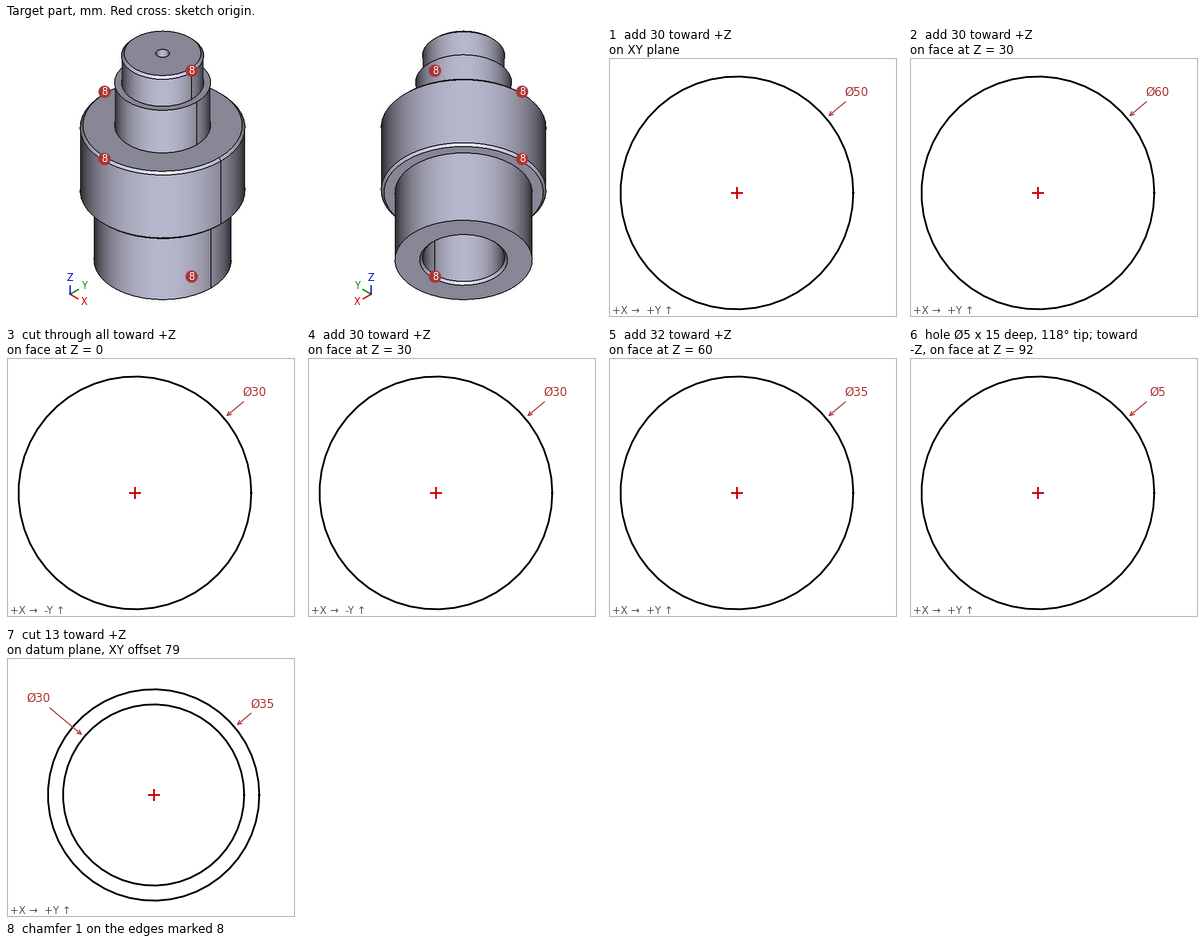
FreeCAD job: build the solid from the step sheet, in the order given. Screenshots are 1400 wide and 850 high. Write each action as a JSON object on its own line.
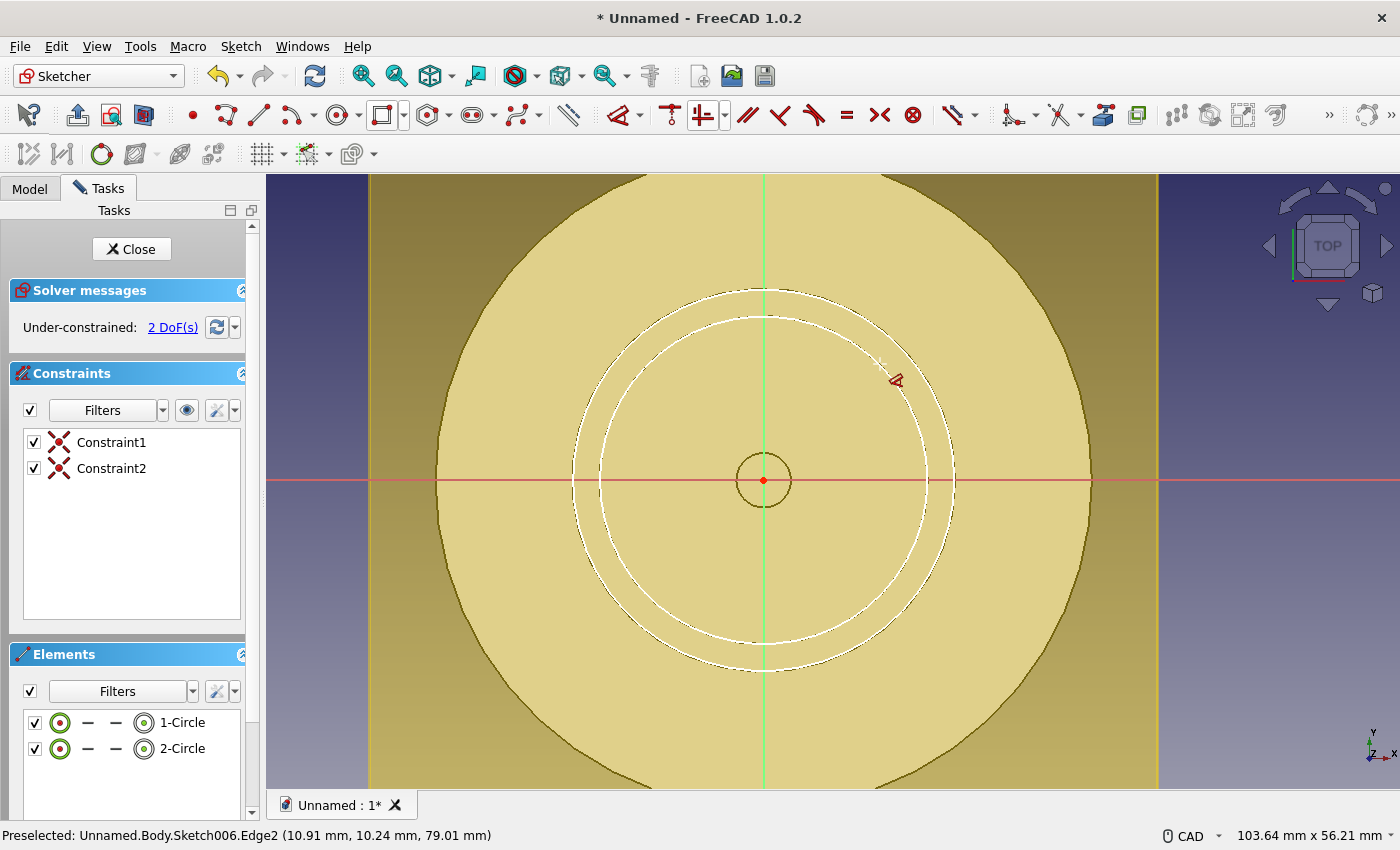
{"action": "left_click", "coordinate": [898, 345]}
{"action": "left_click", "coordinate": [921, 322]}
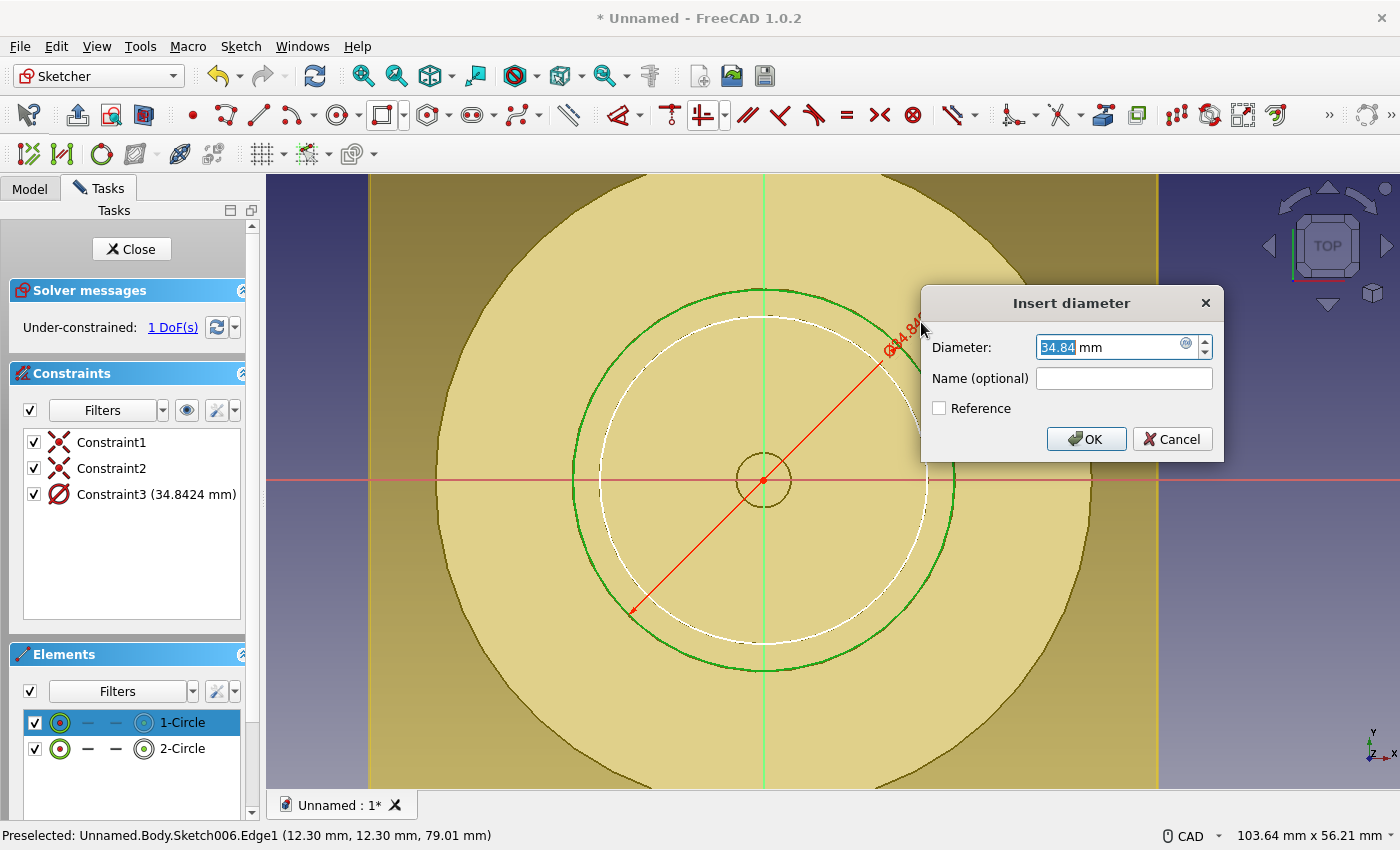
{"action": "type", "text": "35"}
{"action": "key", "text": "Return"}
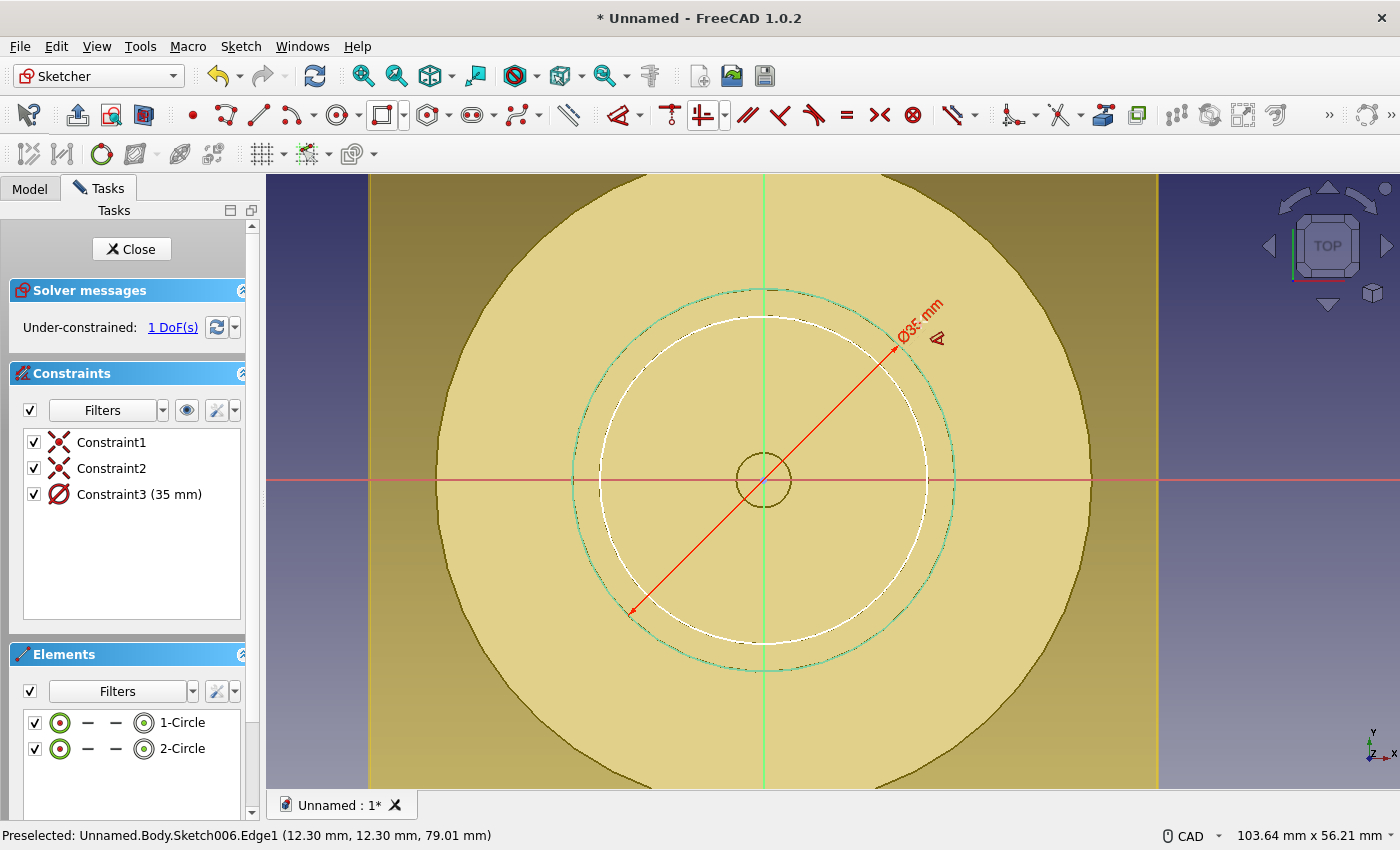
{"action": "left_click", "coordinate": [879, 364]}
{"action": "left_click", "coordinate": [973, 418]}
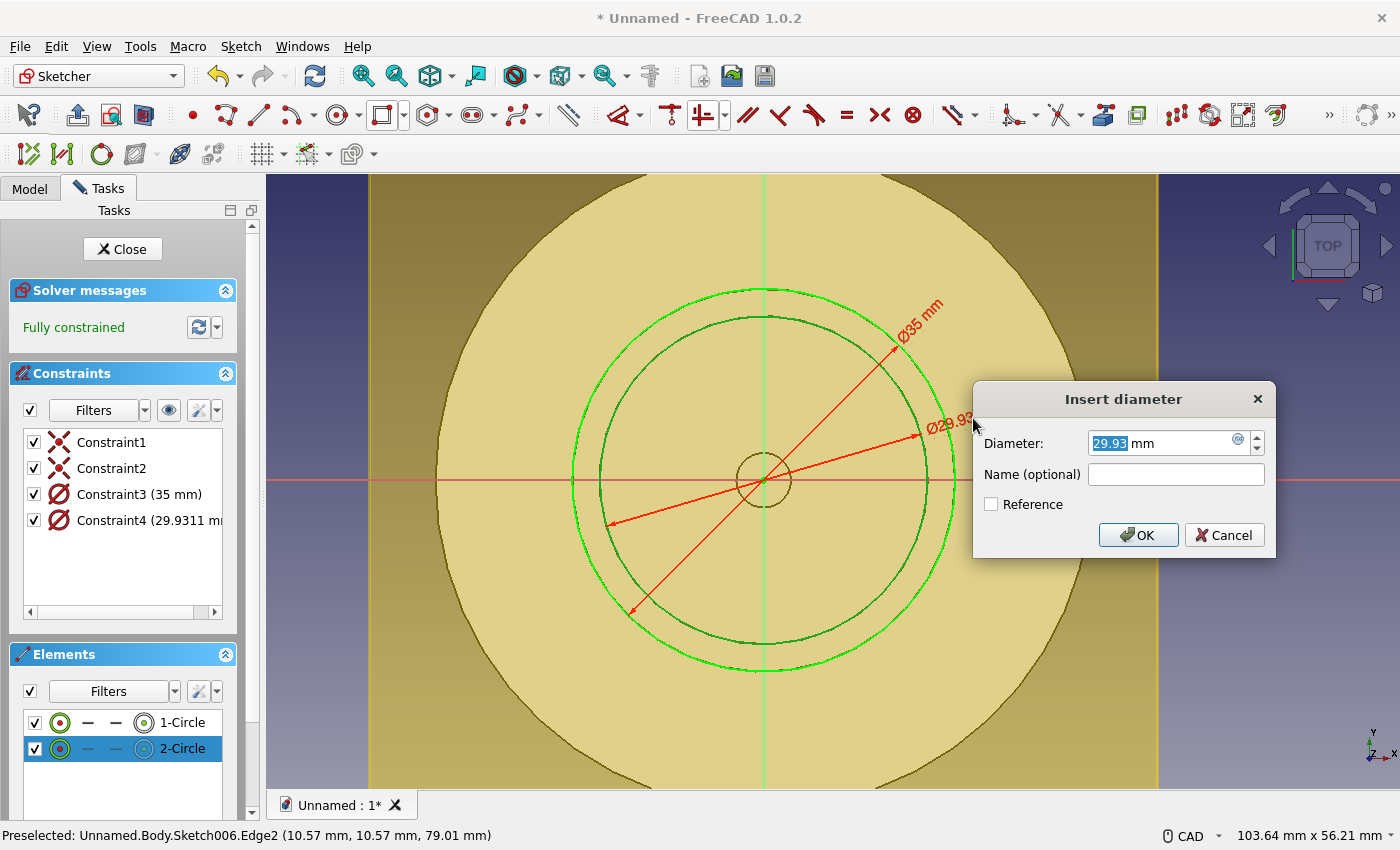
{"action": "type", "text": "30"}
{"action": "key", "text": "Return"}
{"action": "key", "text": "Escape"}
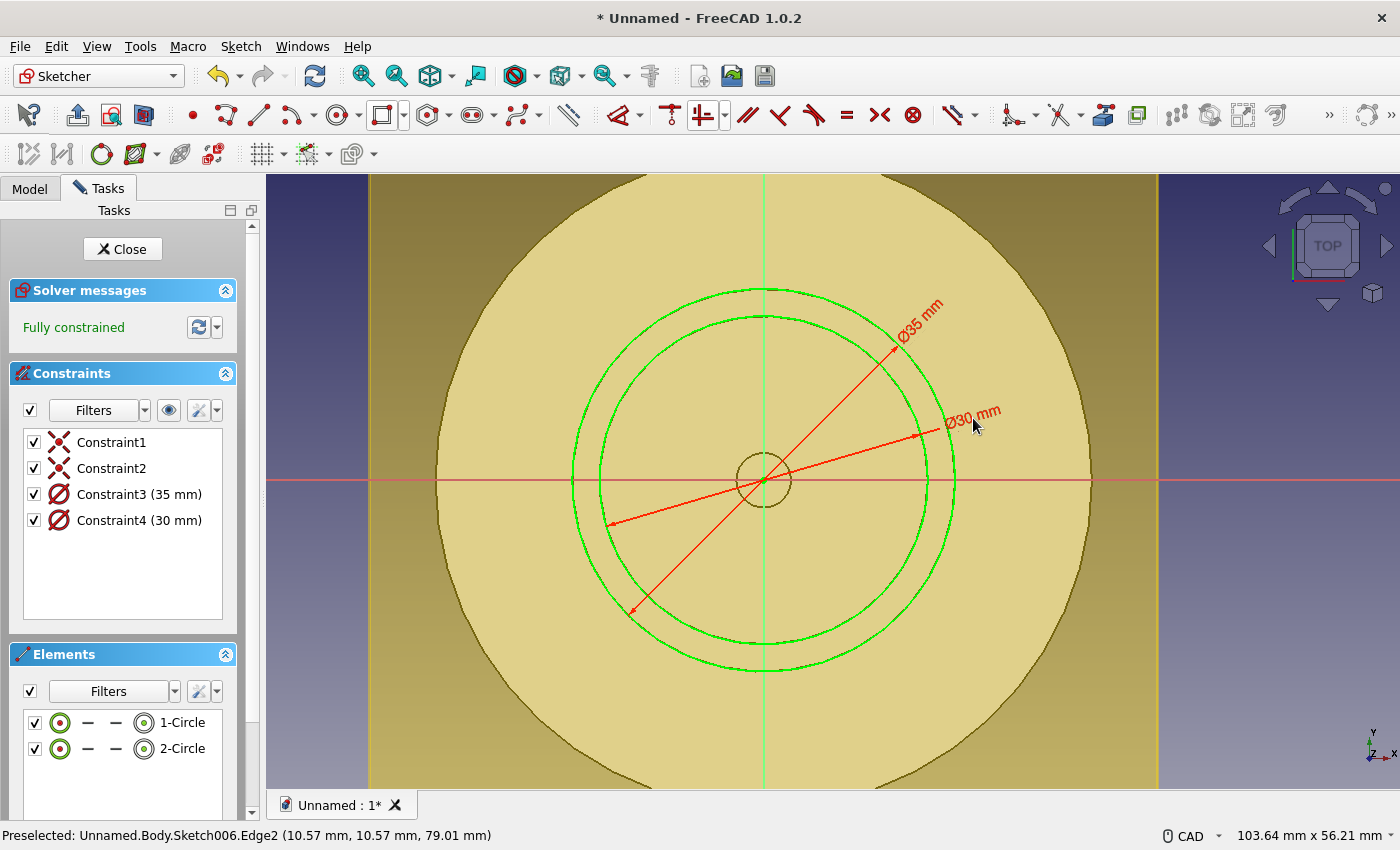
{"action": "left_click", "coordinate": [123, 249]}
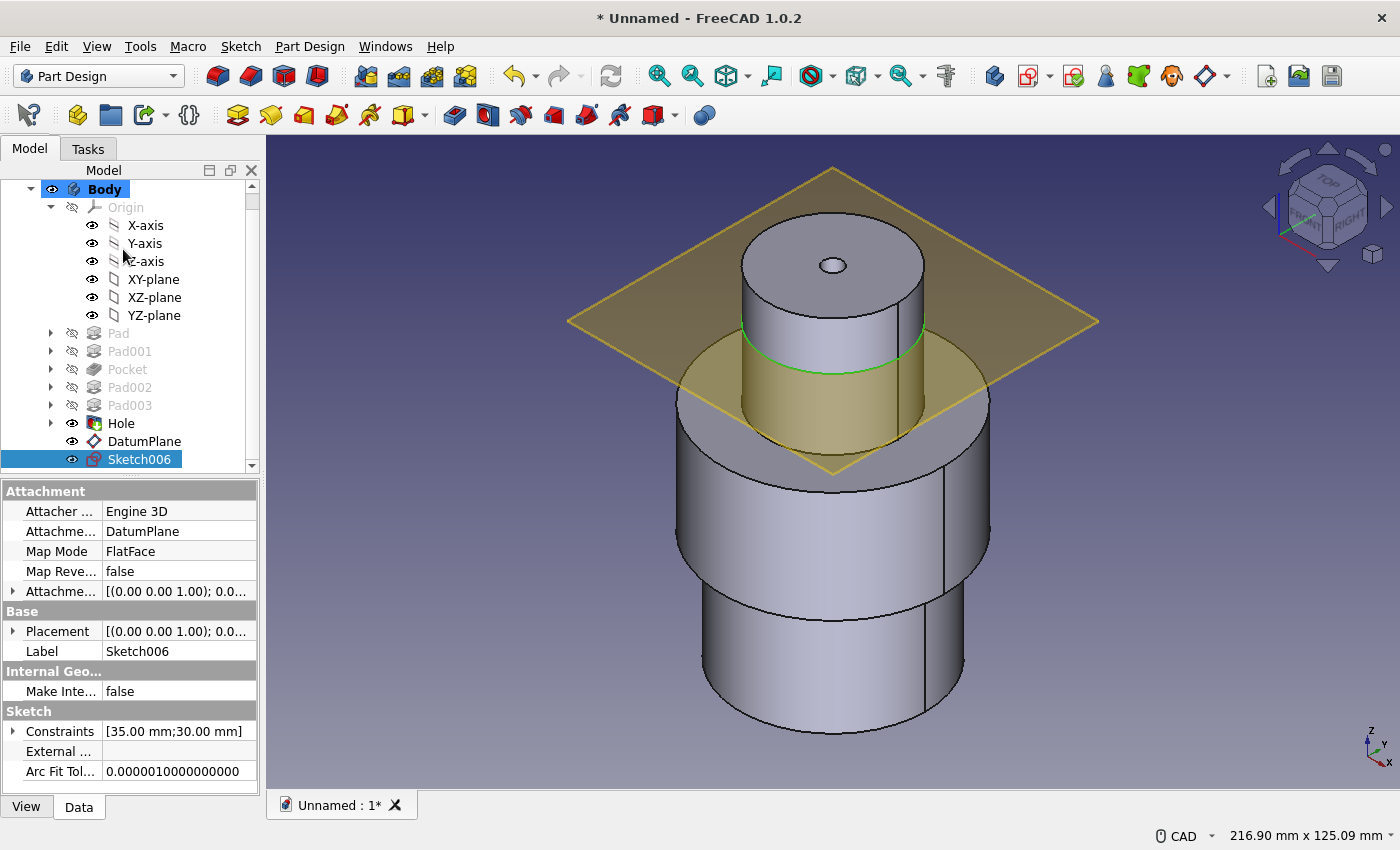
{"action": "left_click", "coordinate": [455, 116]}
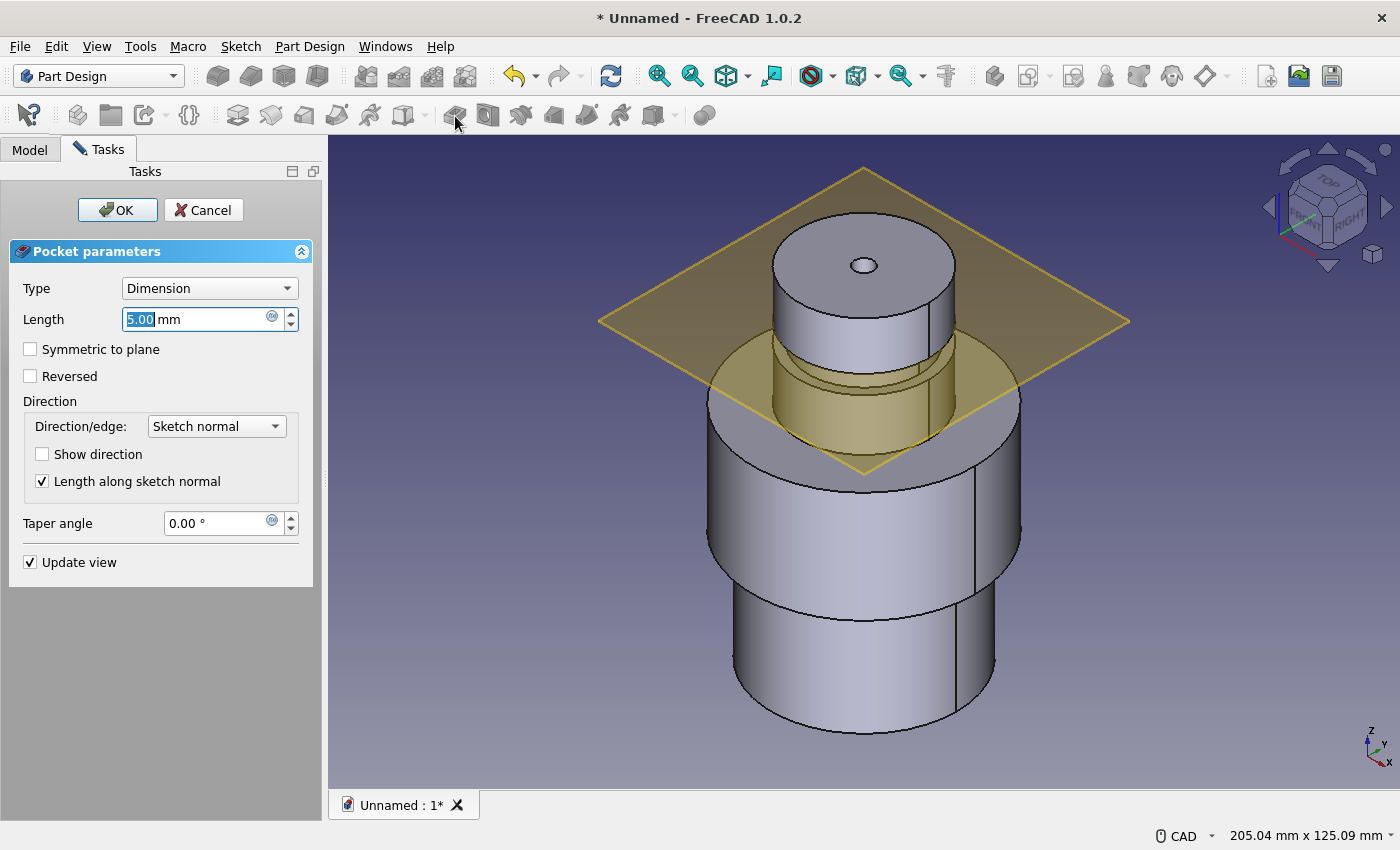
{"action": "type", "text": "13"}
{"action": "key", "text": "Tab"}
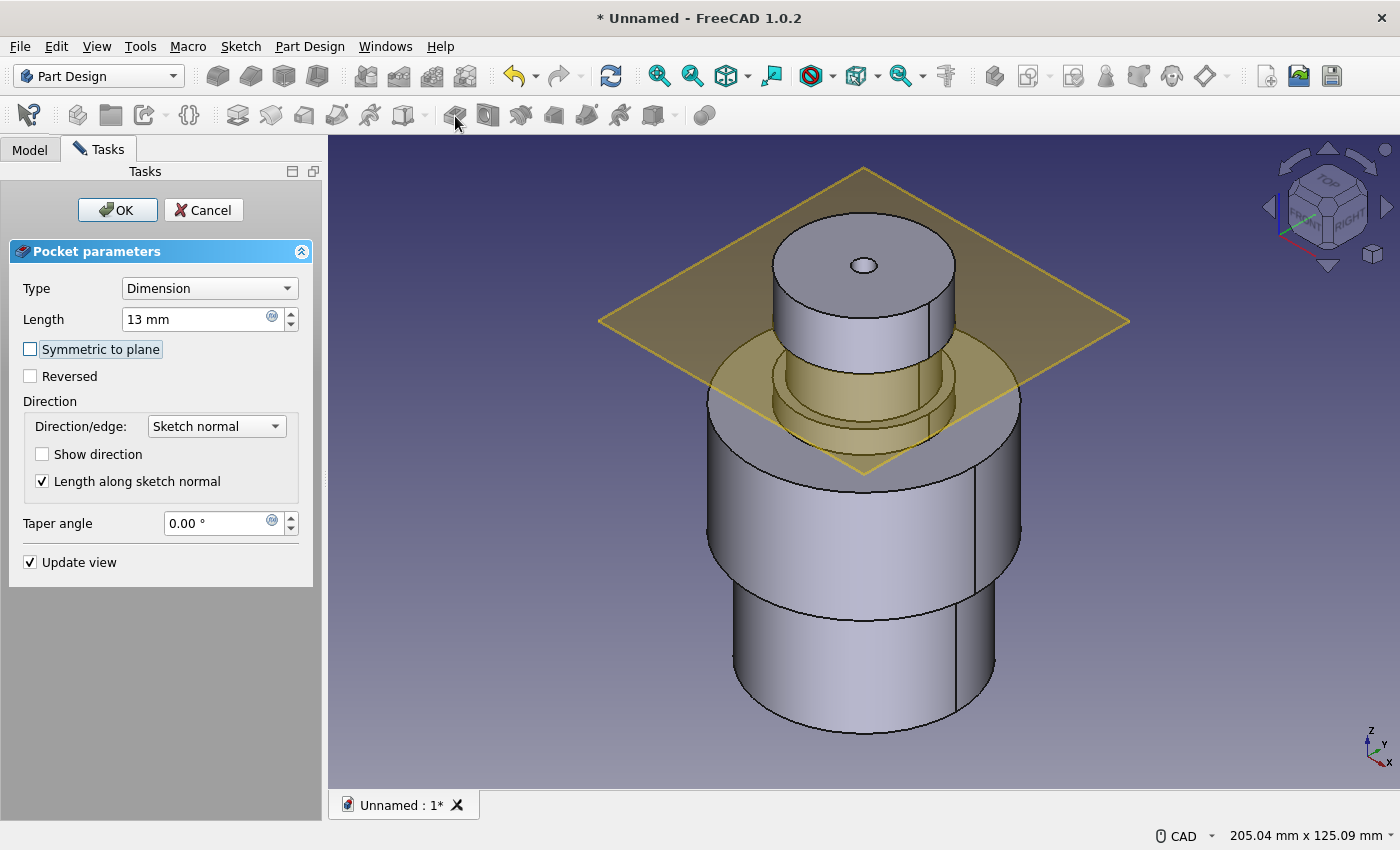
{"action": "left_click", "coordinate": [31, 376]}